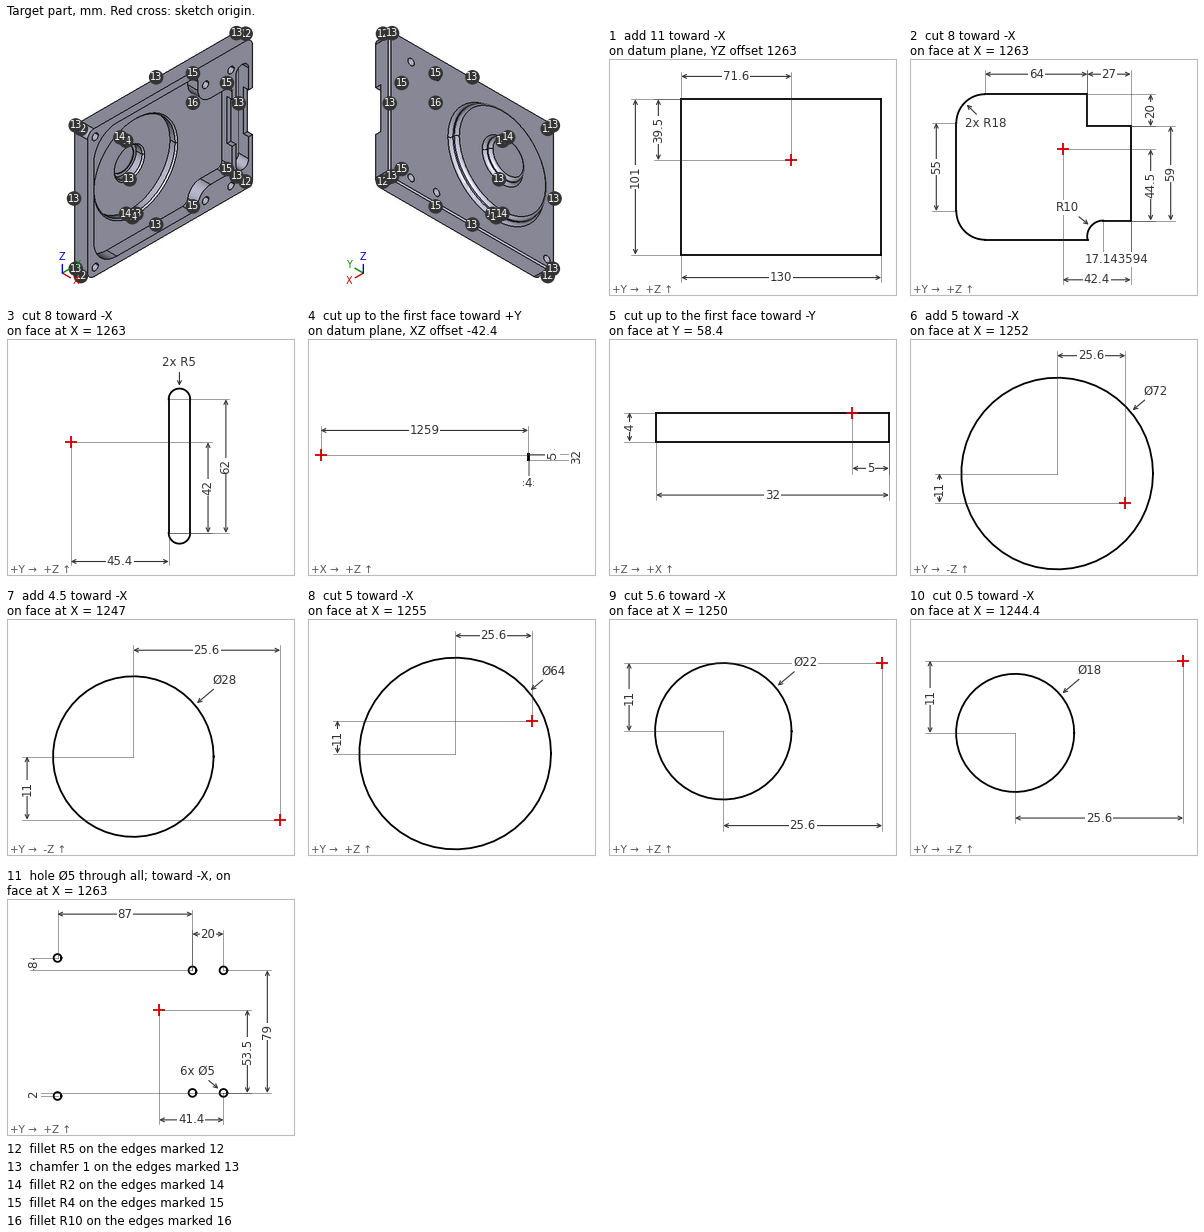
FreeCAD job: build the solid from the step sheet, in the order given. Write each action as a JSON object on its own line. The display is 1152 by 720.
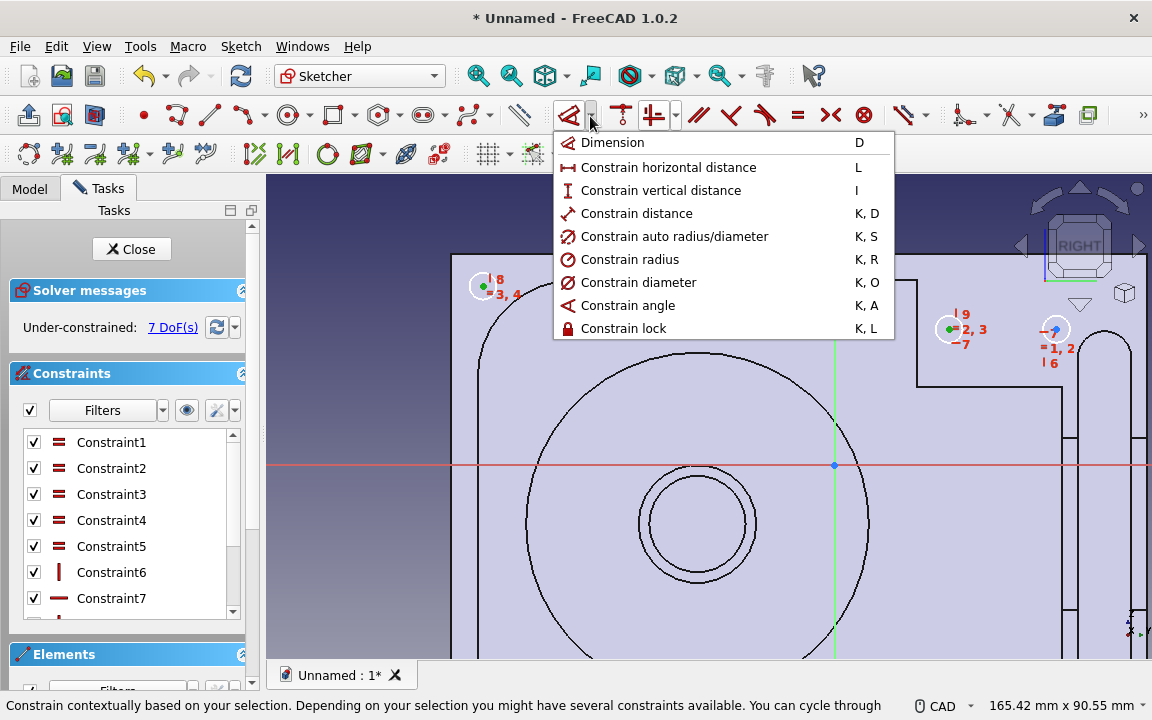
{"action": "left_click", "coordinate": [724, 190]}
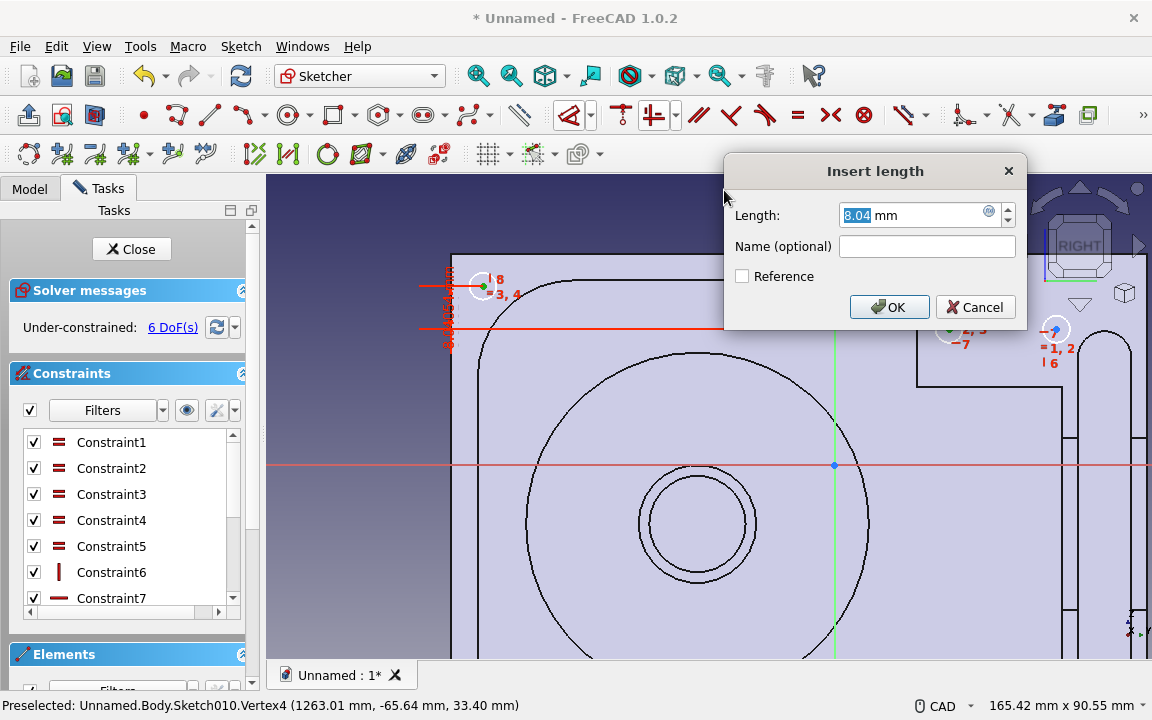
{"action": "type", "text": "8"}
{"action": "key", "text": "Return"}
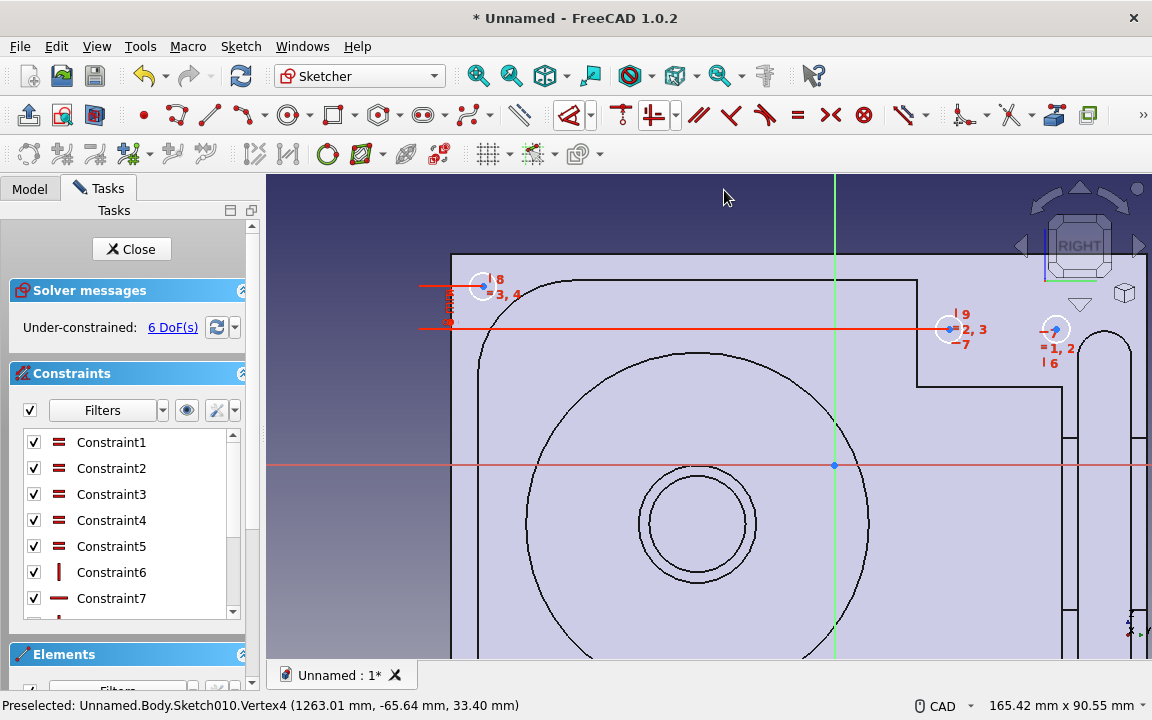
{"action": "scroll", "coordinate": [483, 286], "scroll_direction": "down", "scroll_amount": 3}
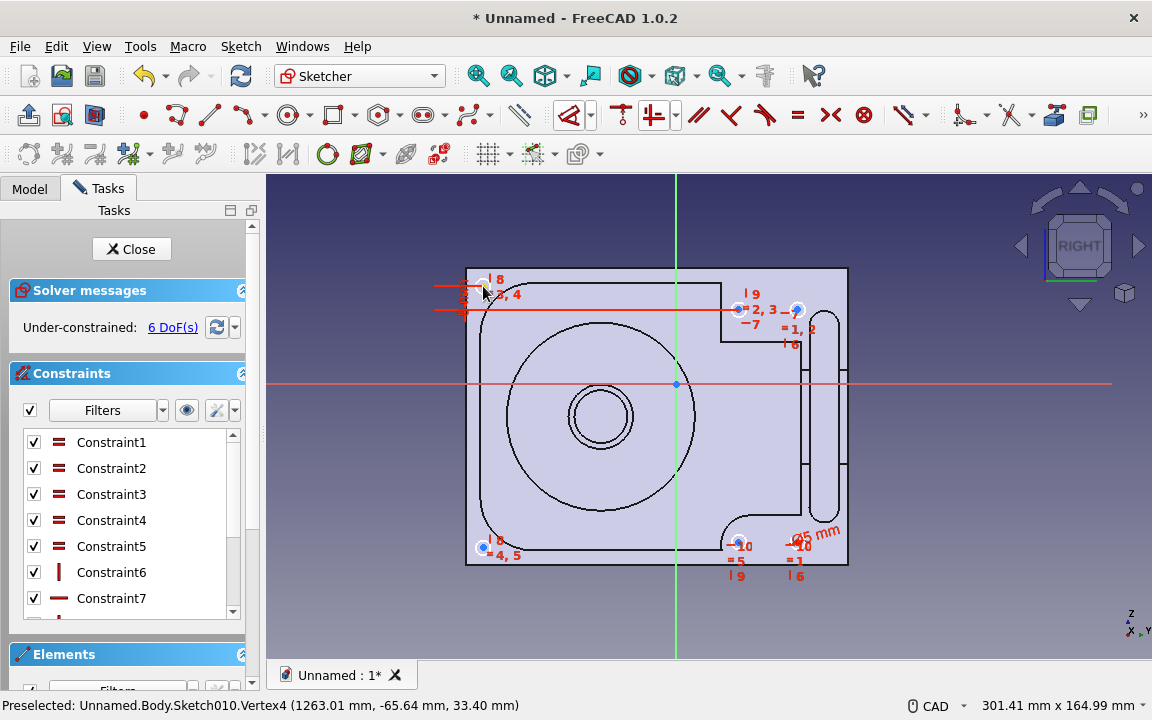
{"action": "scroll", "coordinate": [798, 542], "scroll_direction": "up", "scroll_amount": 10}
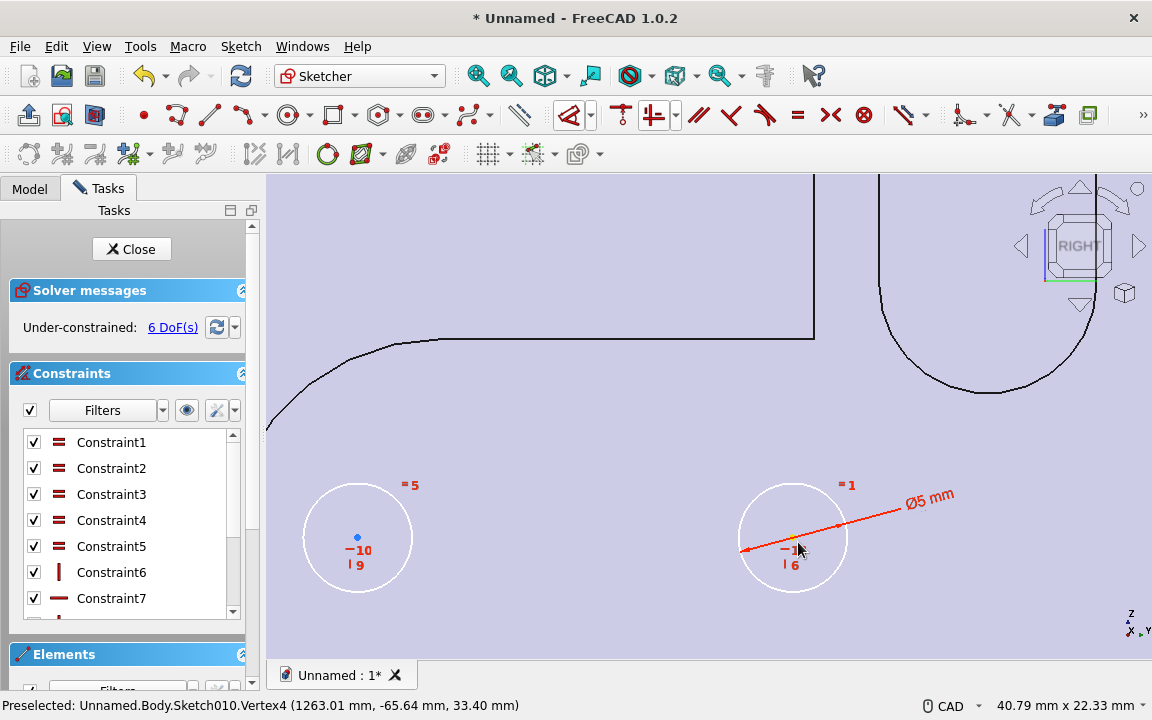
{"action": "left_click", "coordinate": [793, 538]}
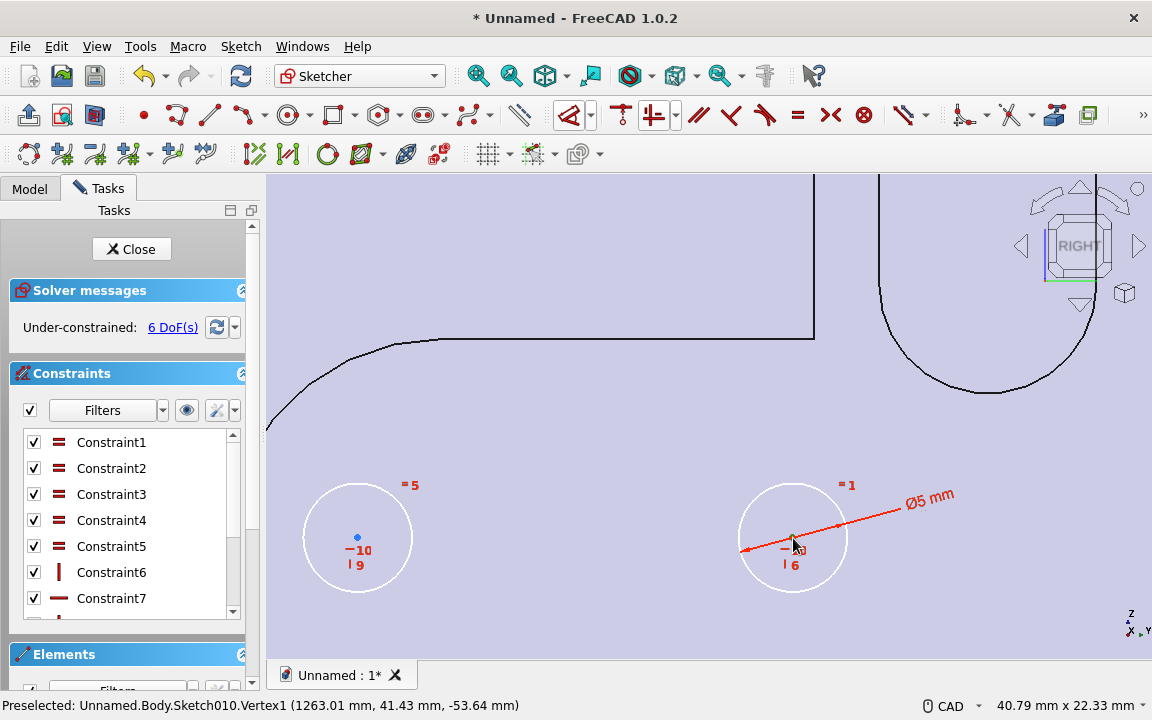
{"action": "scroll", "coordinate": [799, 542], "scroll_direction": "down", "scroll_amount": 10}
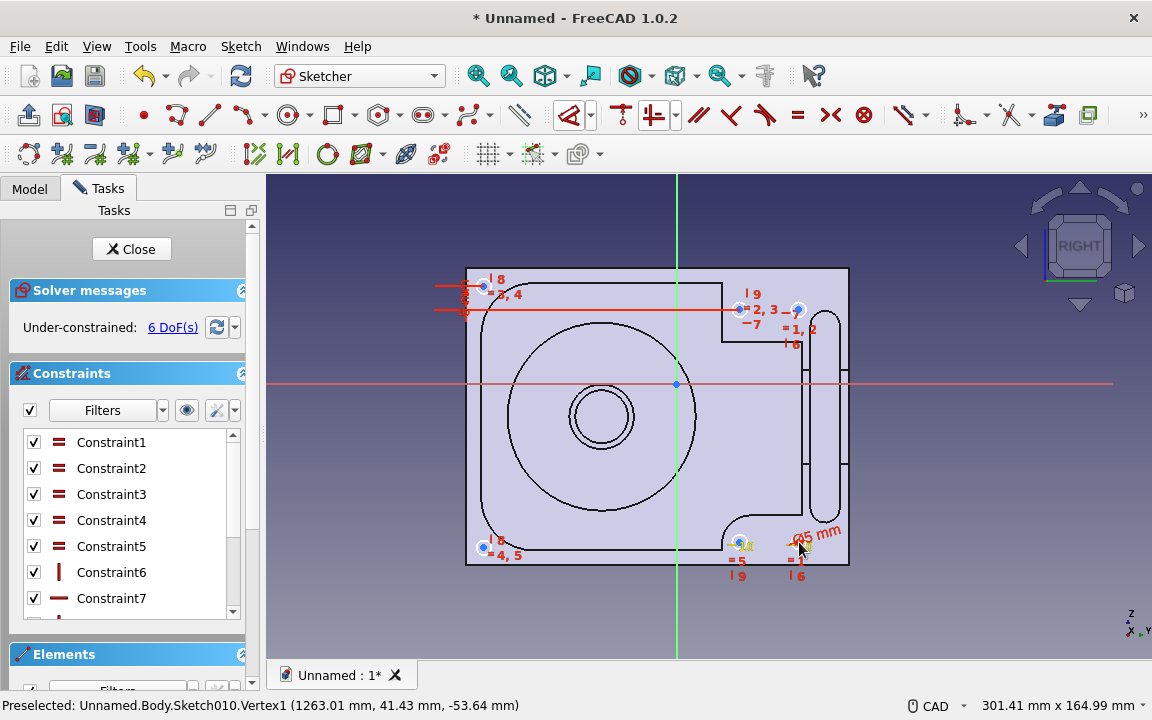
{"action": "scroll", "coordinate": [484, 548], "scroll_direction": "up", "scroll_amount": 10}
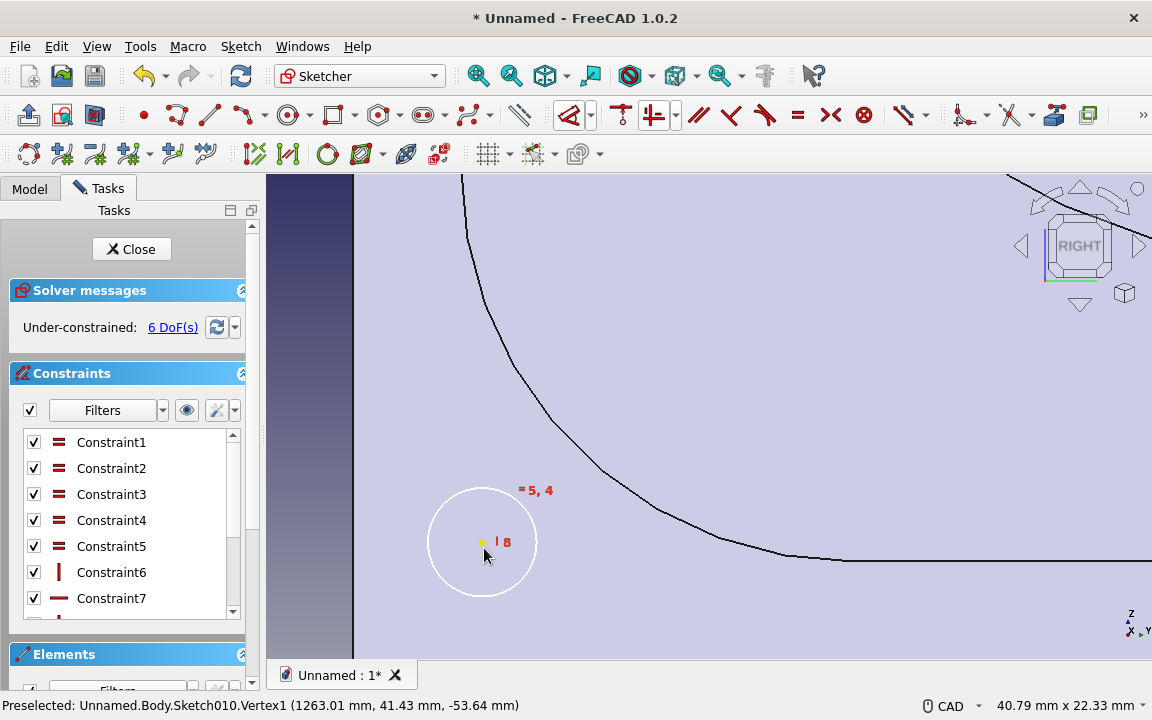
{"action": "left_click", "coordinate": [482, 542]}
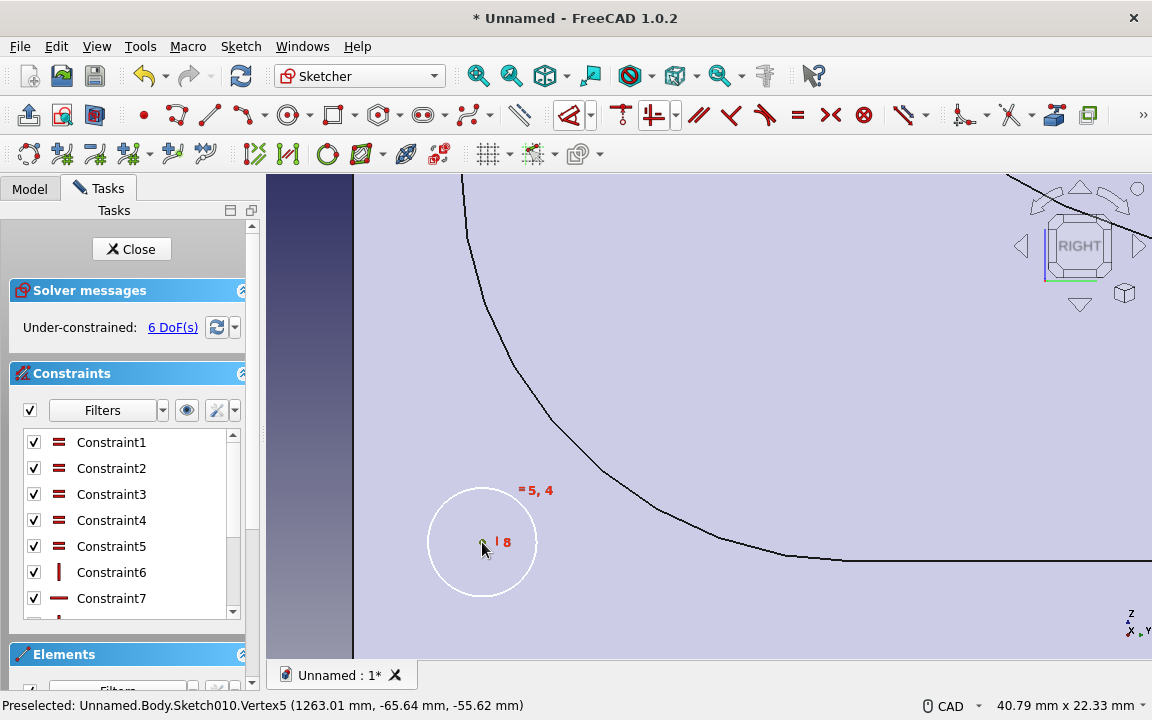
{"action": "left_click", "coordinate": [590, 116]}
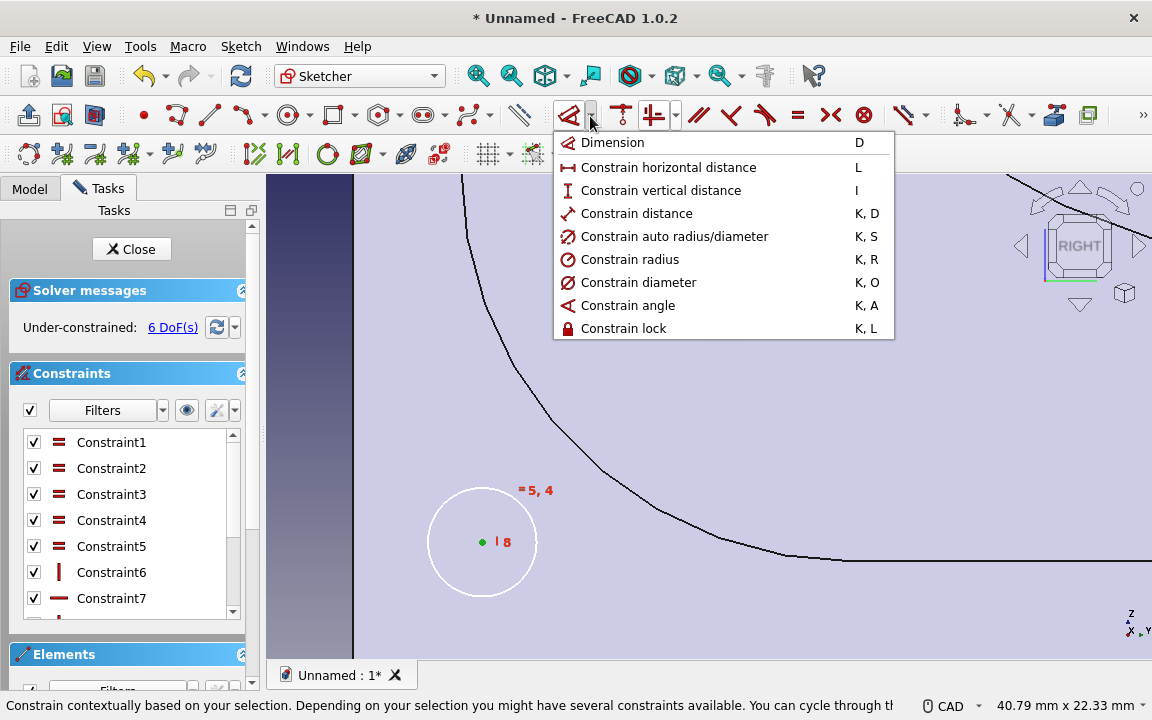
{"action": "left_click", "coordinate": [724, 190]}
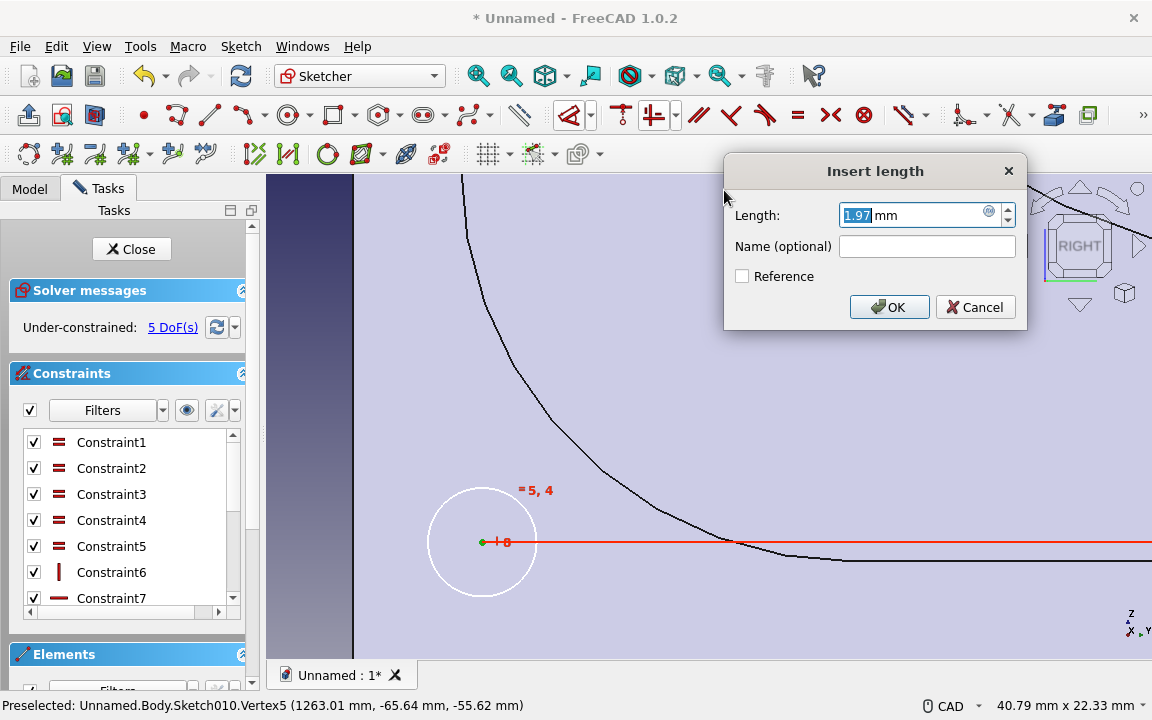
{"action": "type", "text": "2"}
{"action": "key", "text": "Return"}